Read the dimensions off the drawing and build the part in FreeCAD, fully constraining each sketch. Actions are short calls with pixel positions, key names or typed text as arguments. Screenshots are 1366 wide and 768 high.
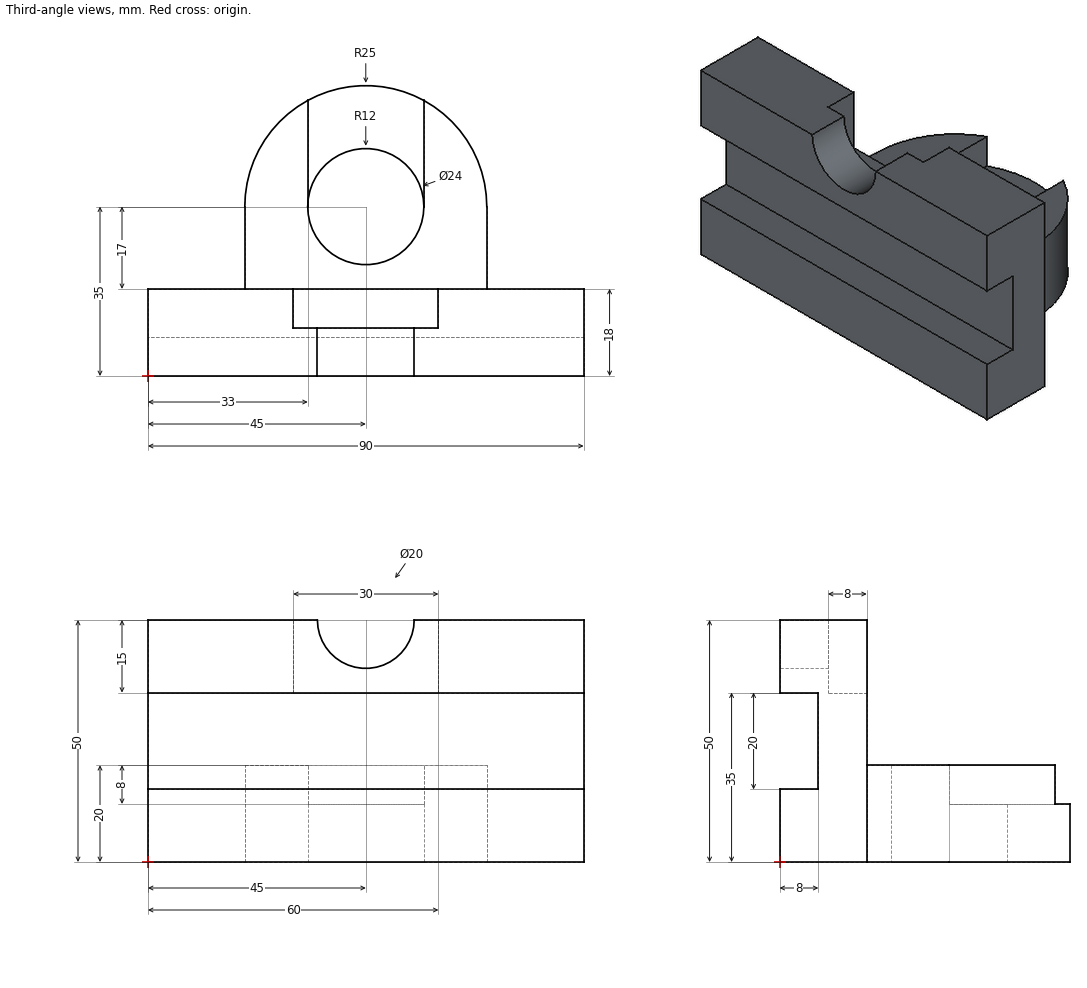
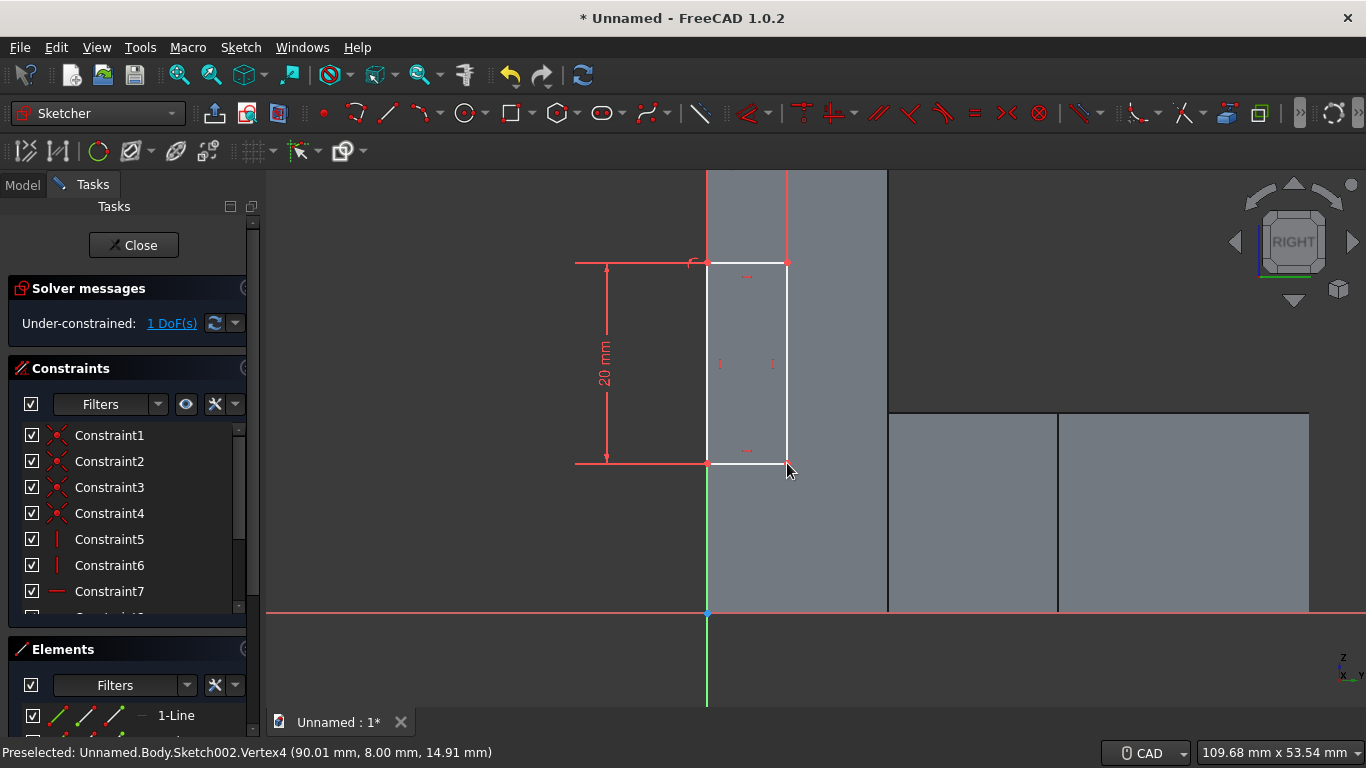
key(d)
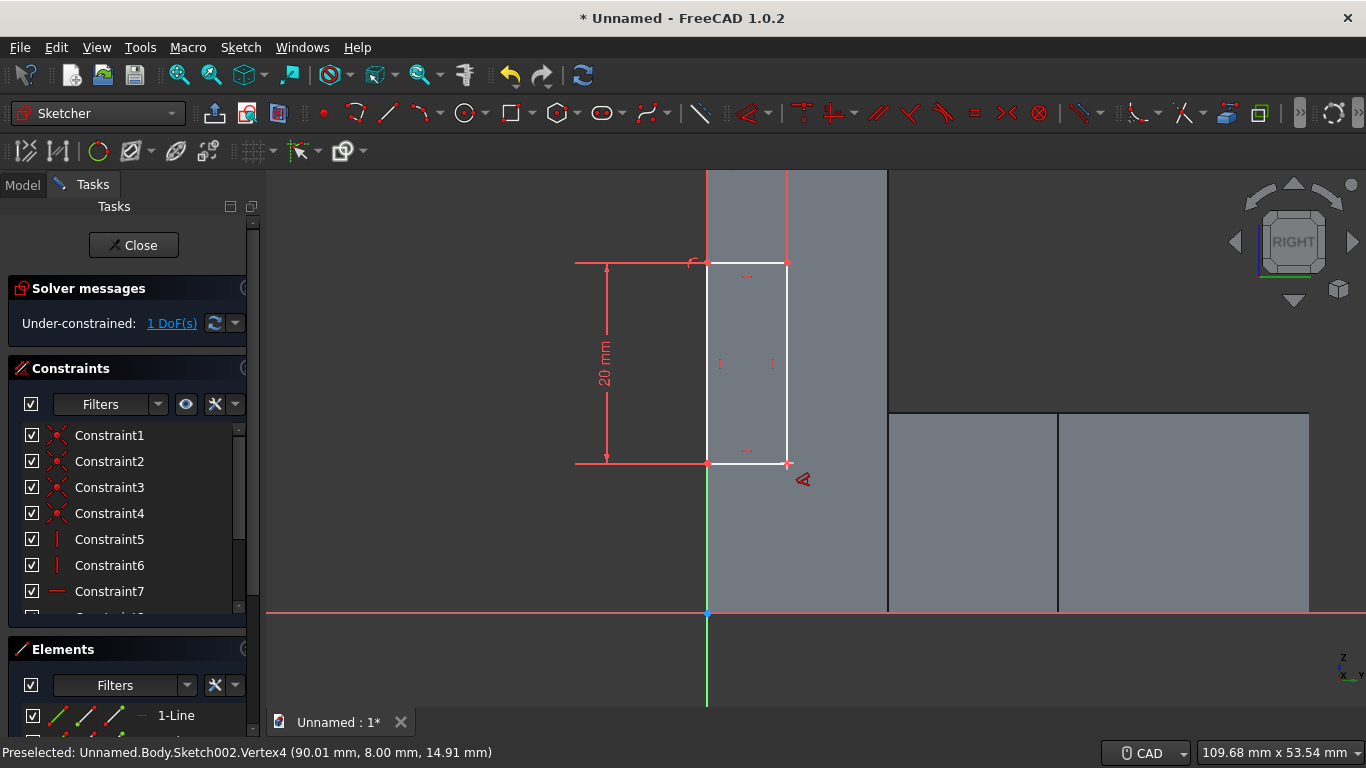
click(707, 263)
click(673, 438)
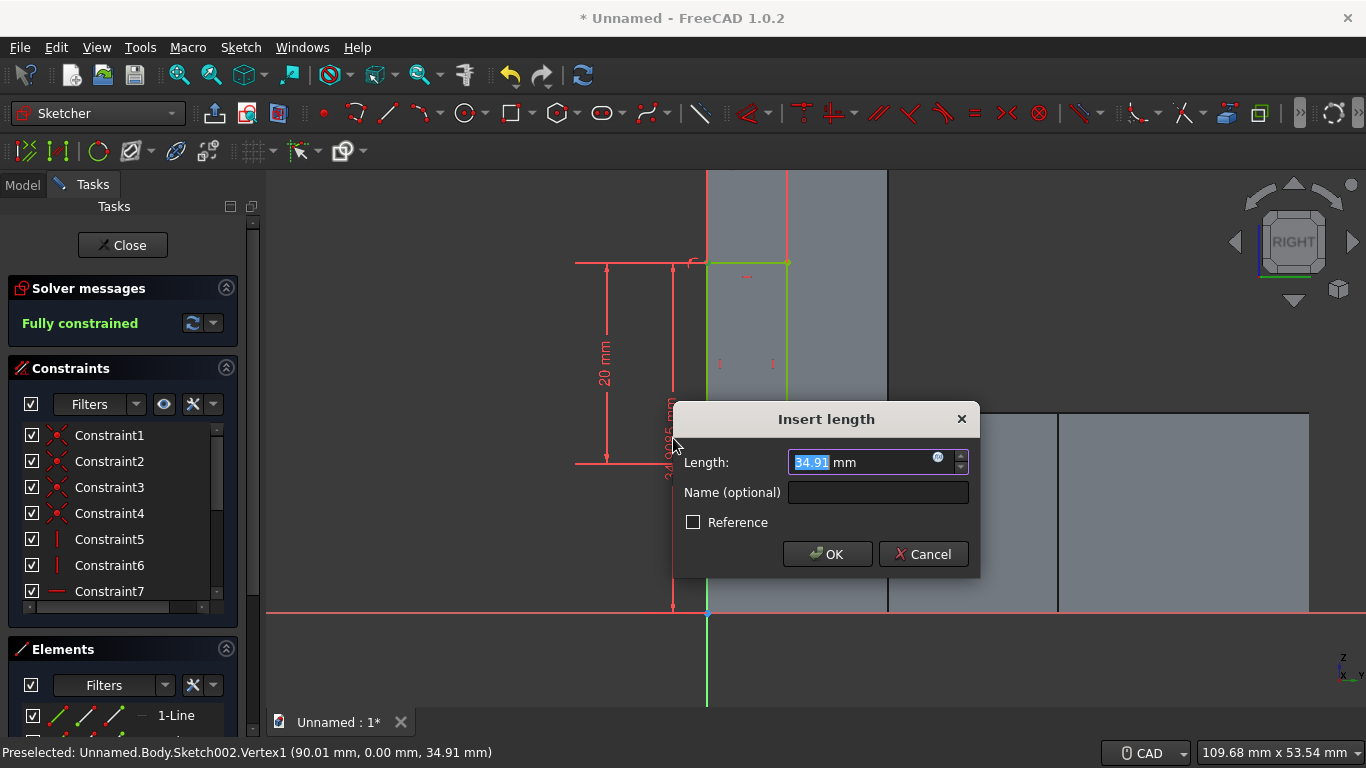
text(35)
key(Return)
key(Escape)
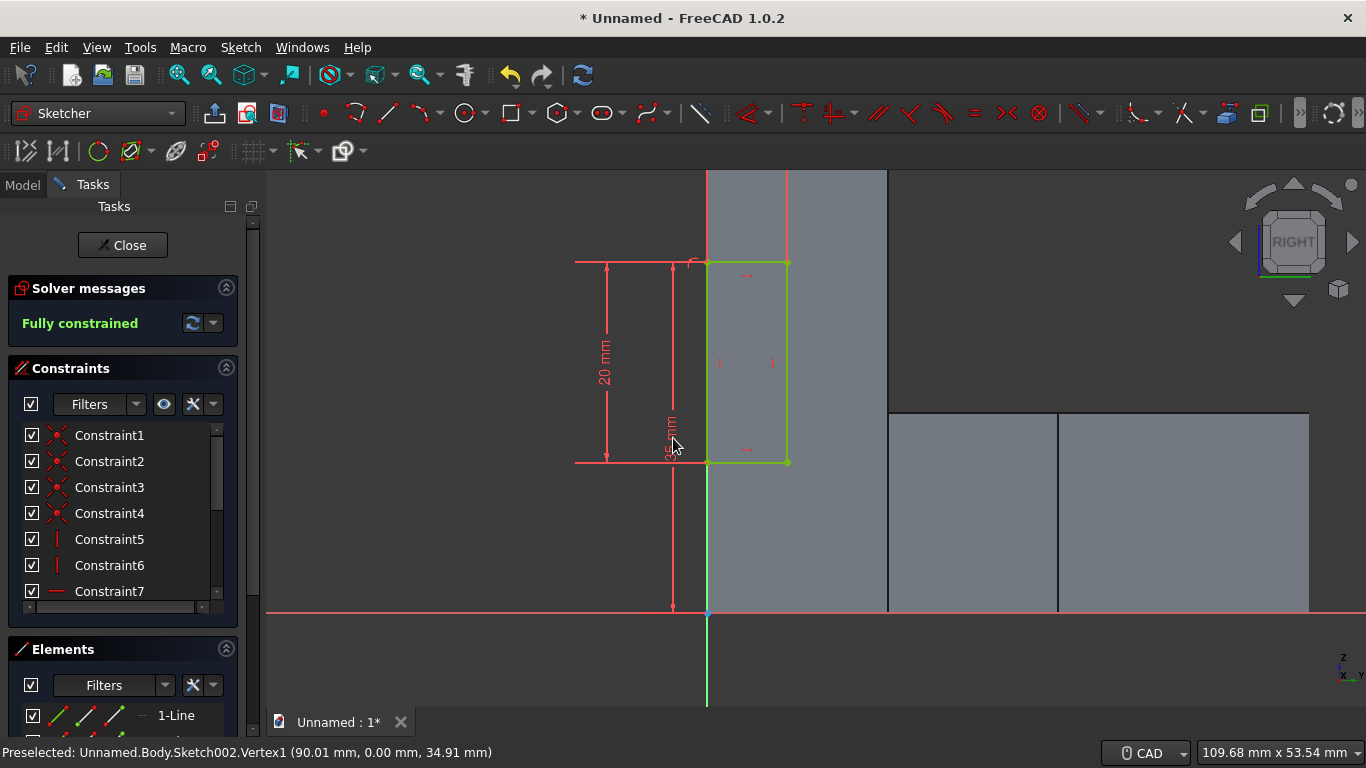
click(123, 245)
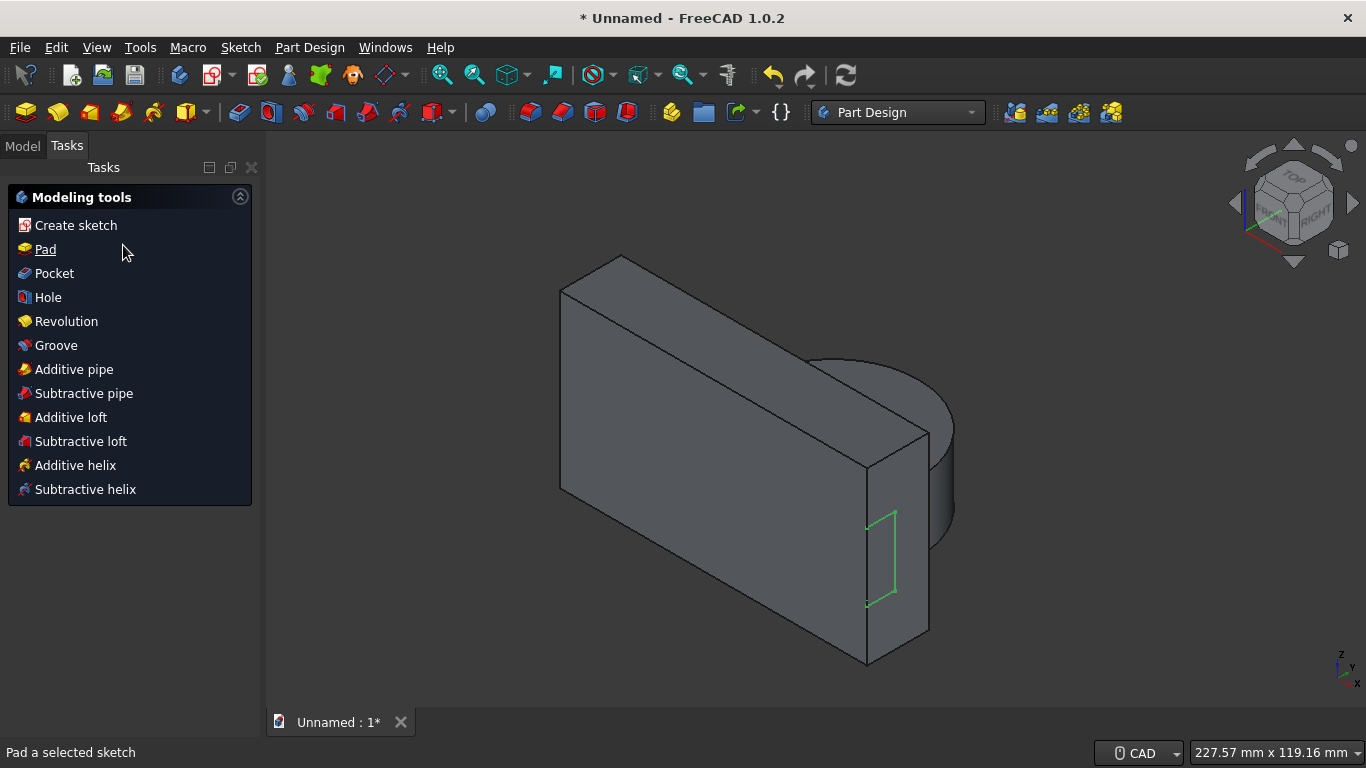
click(240, 112)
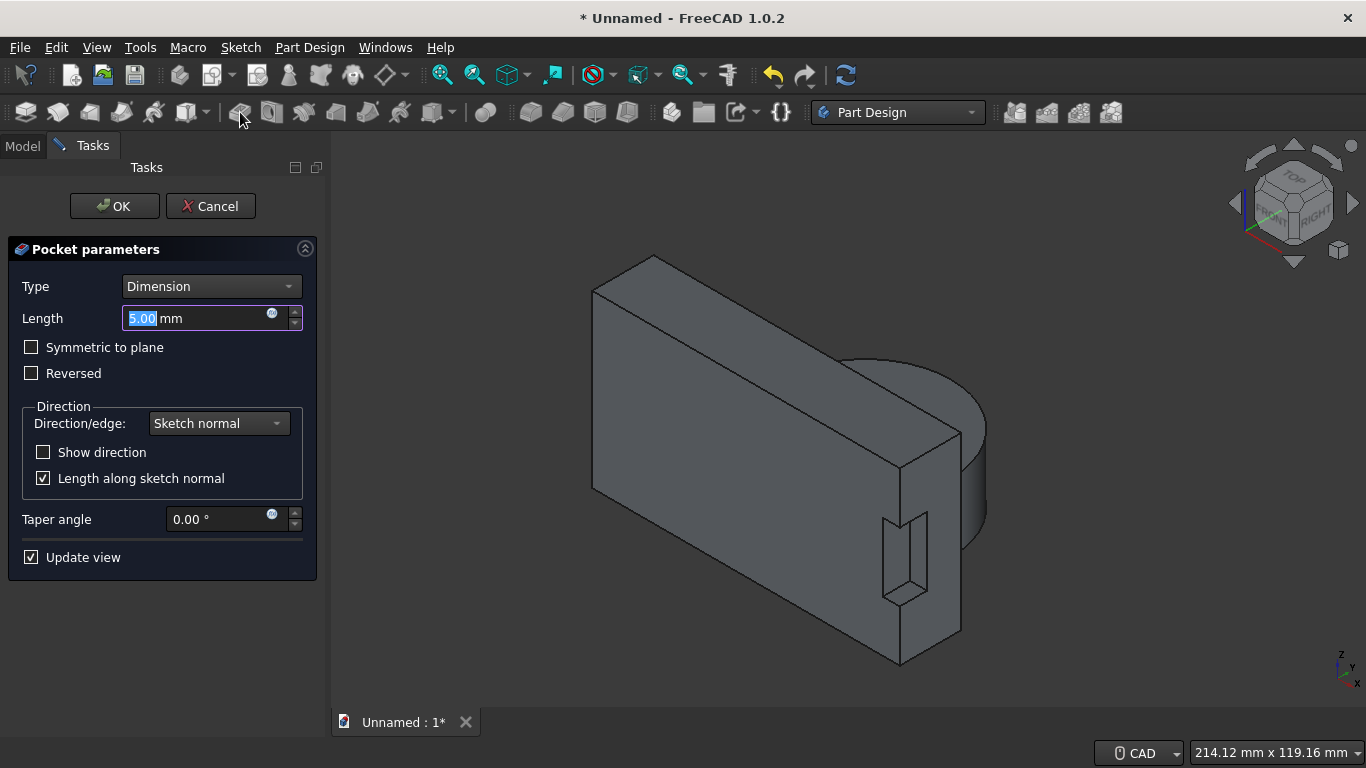
click(212, 286)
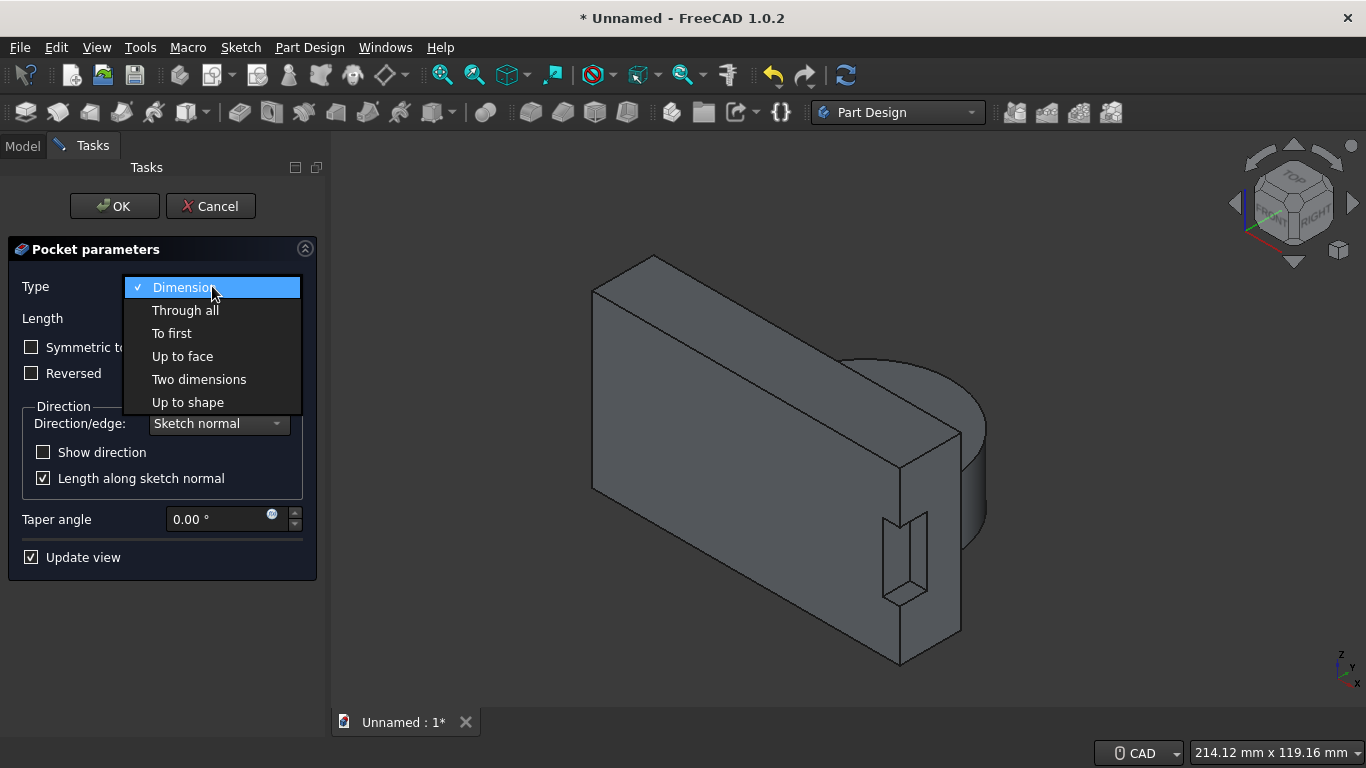
click(212, 310)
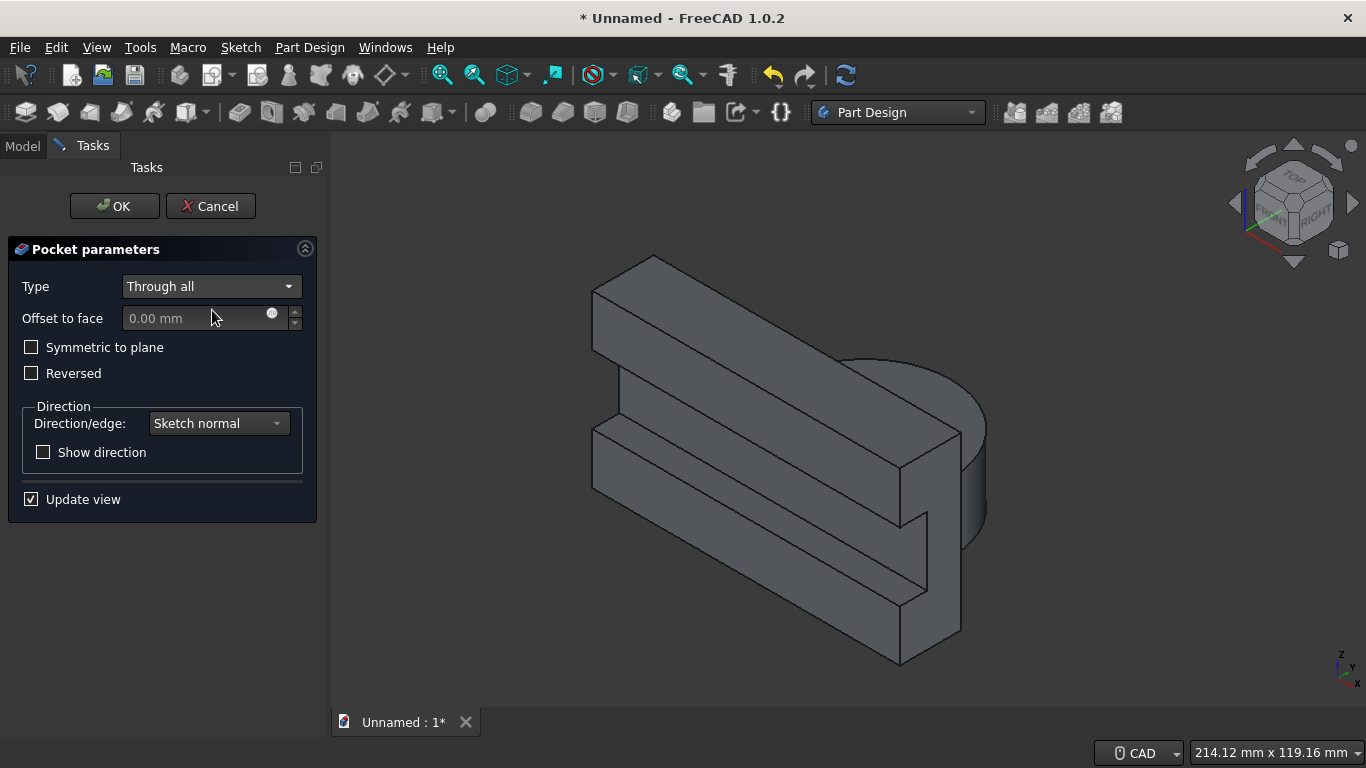
click(115, 206)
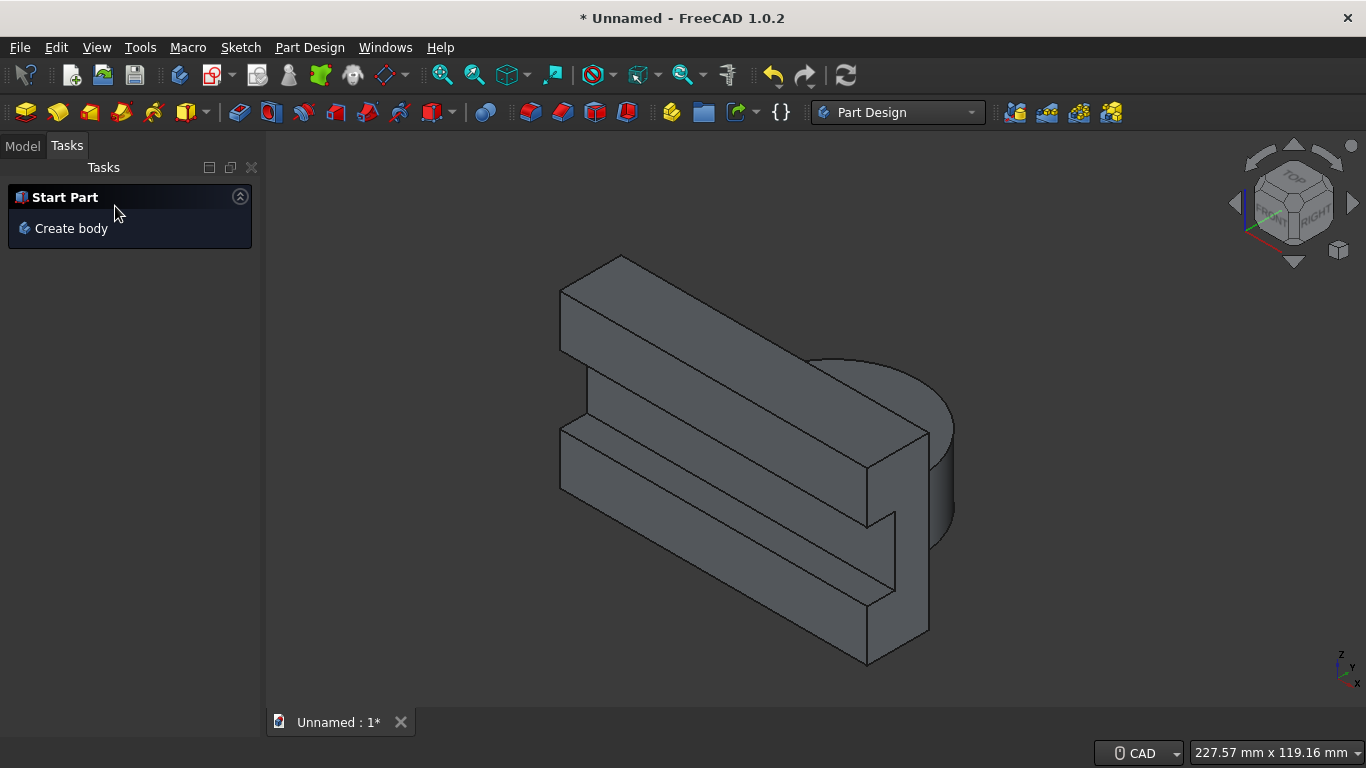
click(23, 145)